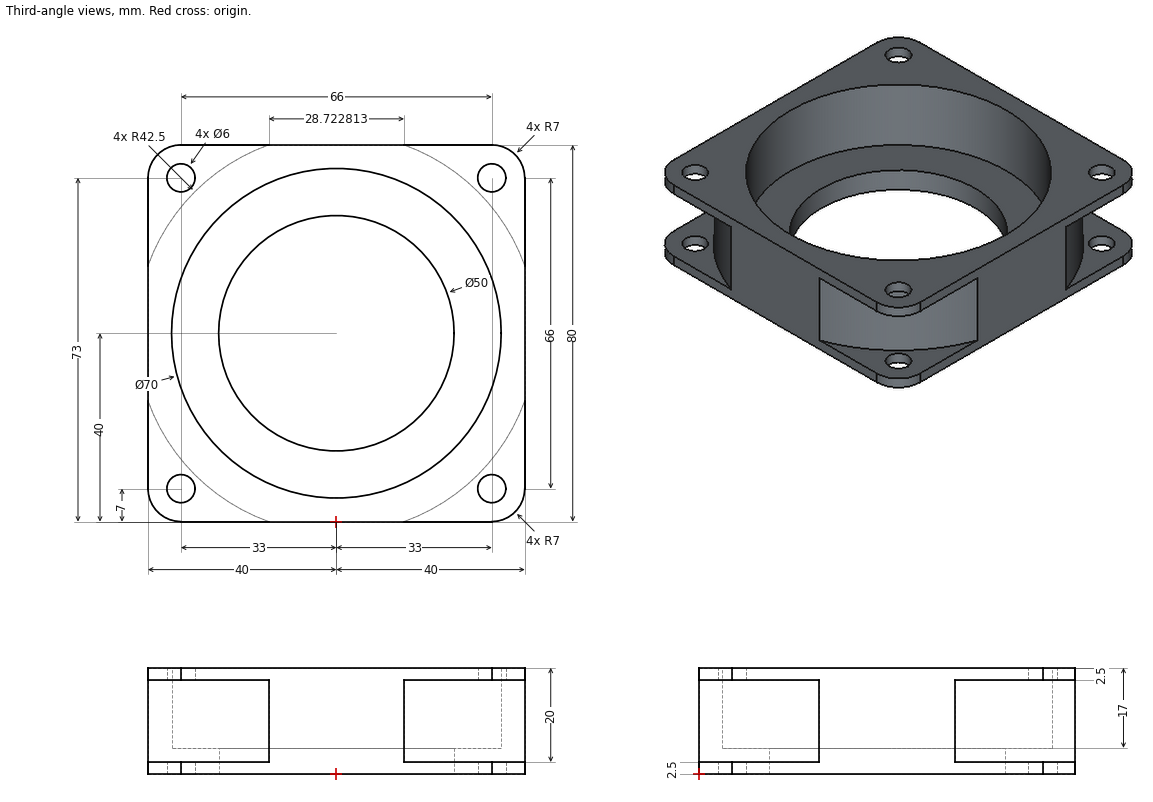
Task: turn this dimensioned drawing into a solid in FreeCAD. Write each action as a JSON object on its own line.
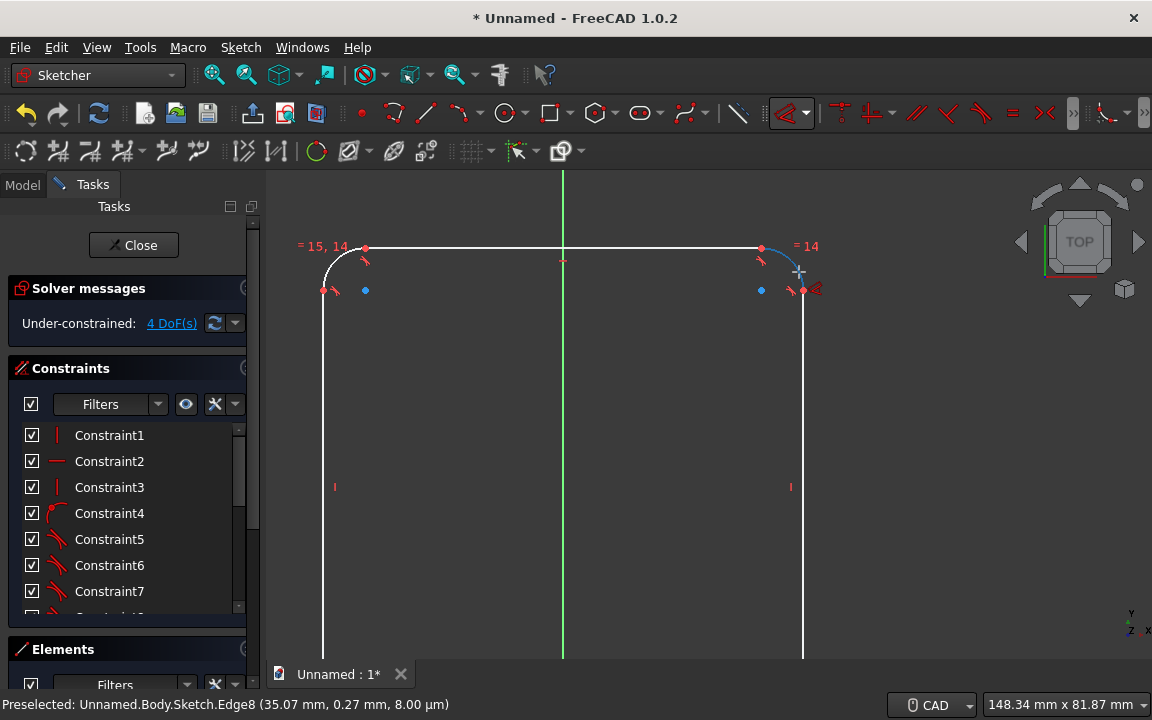
{"action": "left_click", "coordinate": [799, 271]}
{"action": "left_click", "coordinate": [827, 256]}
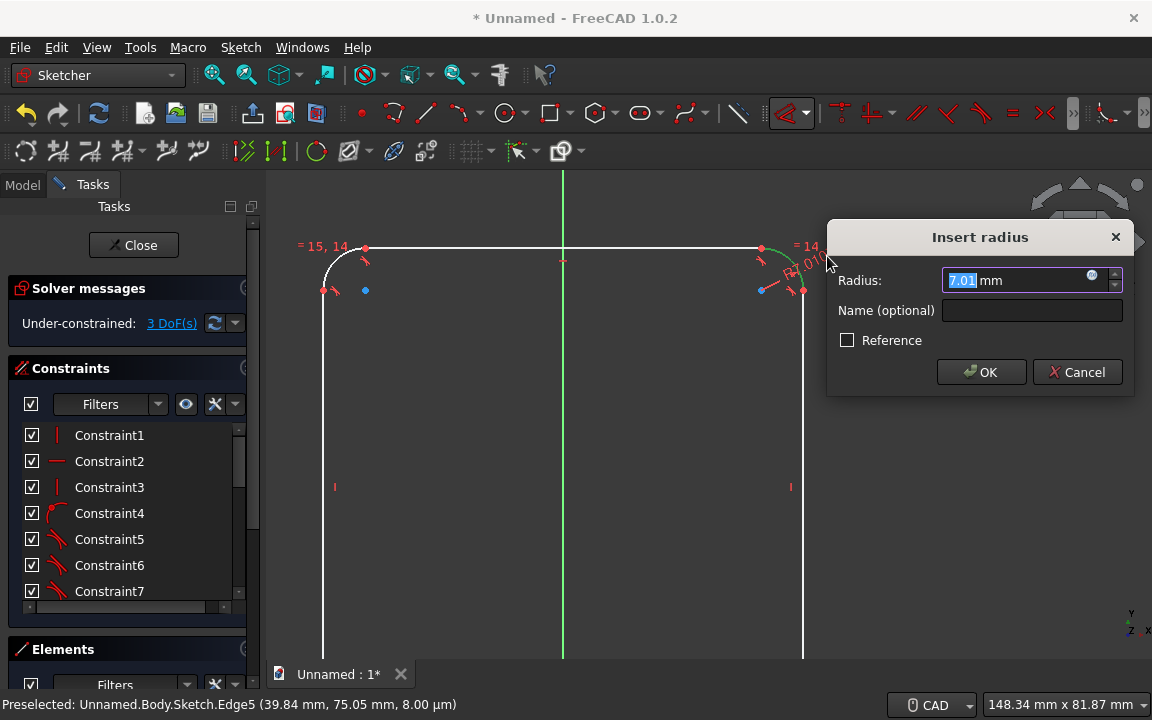
{"action": "type", "text": "7"}
{"action": "key", "text": "Return"}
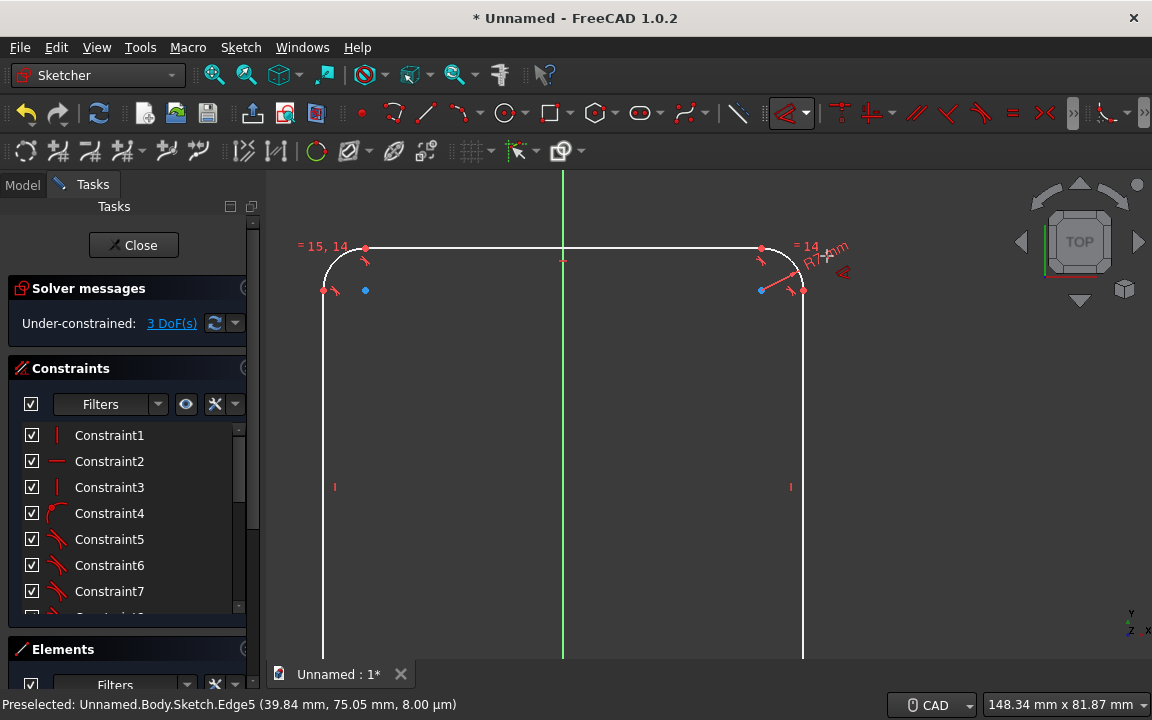
{"action": "left_click", "coordinate": [803, 565]}
{"action": "left_click", "coordinate": [837, 461]}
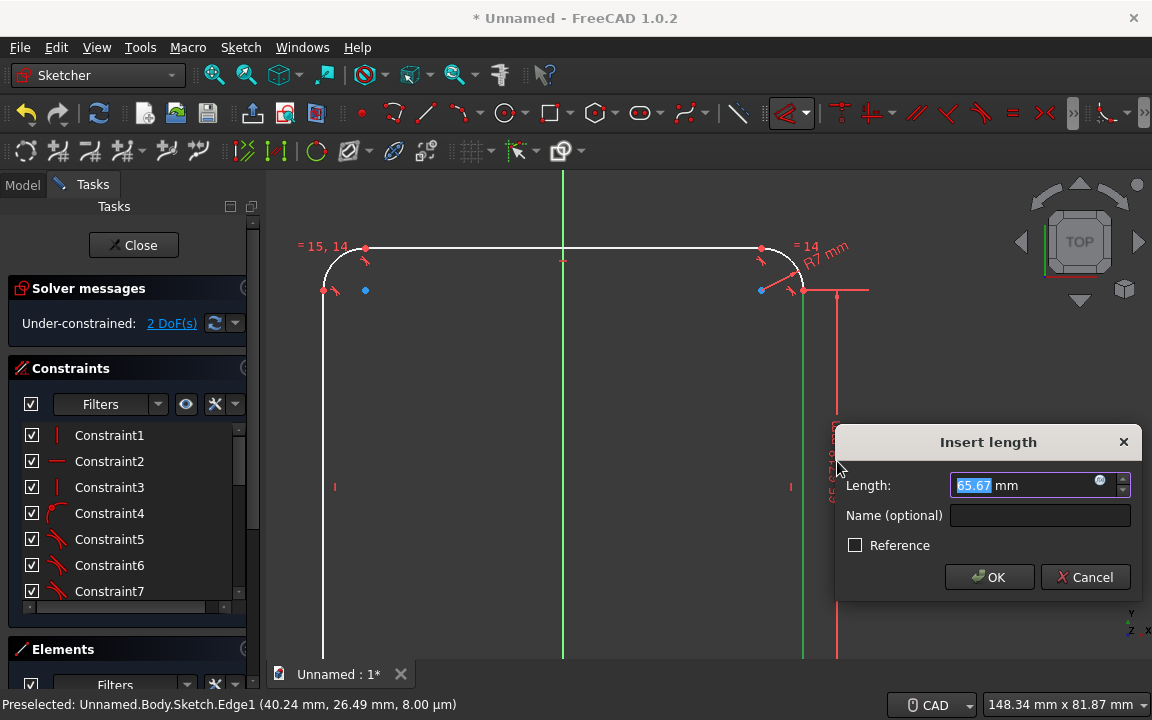
{"action": "type", "text": "66"}
{"action": "key", "text": "Return"}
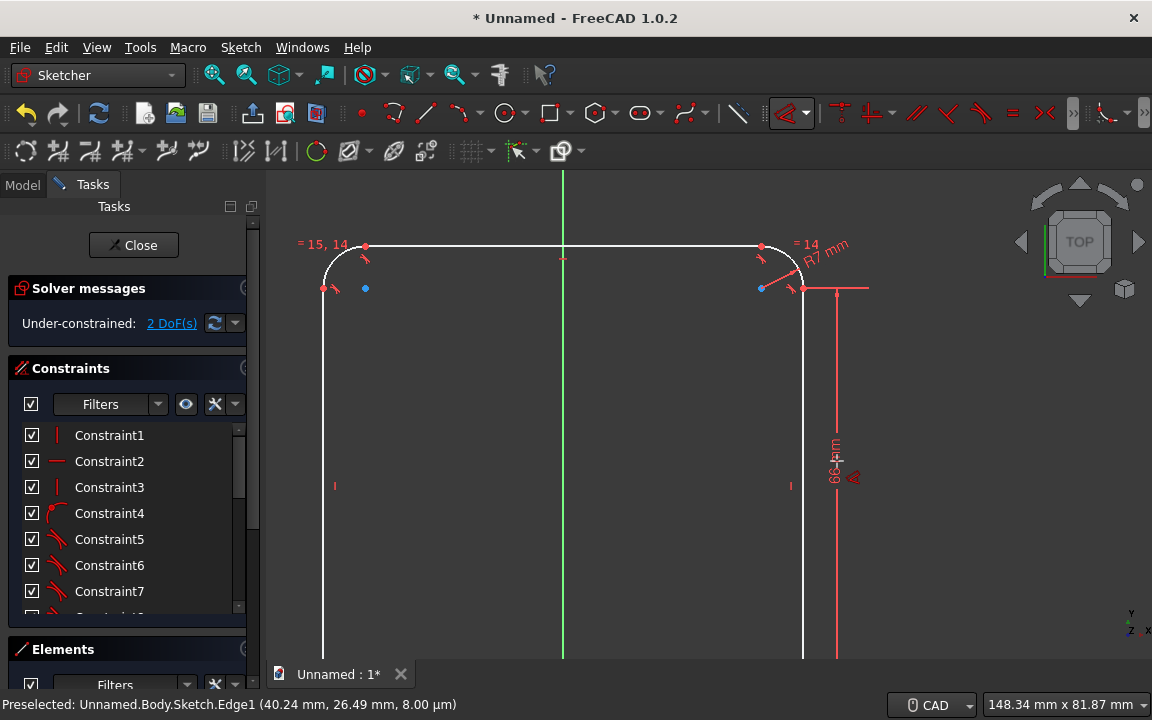
{"action": "left_click", "coordinate": [643, 246]}
{"action": "left_click", "coordinate": [472, 212]}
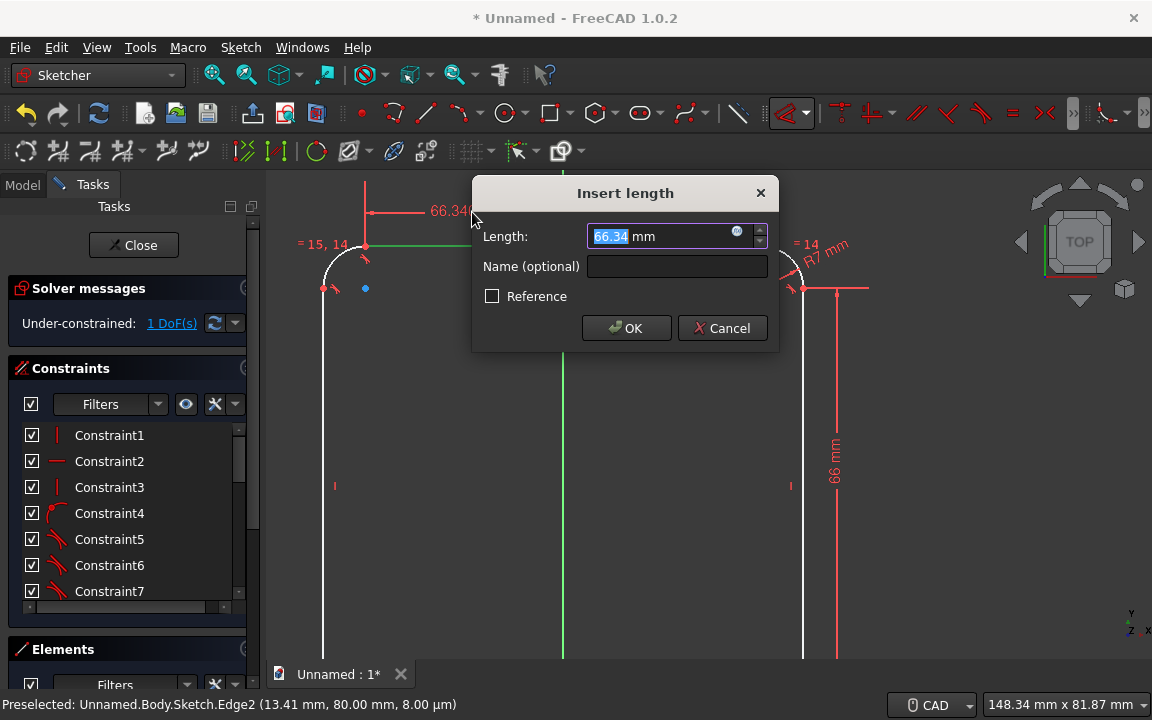
{"action": "type", "text": "66"}
{"action": "key", "text": "Return"}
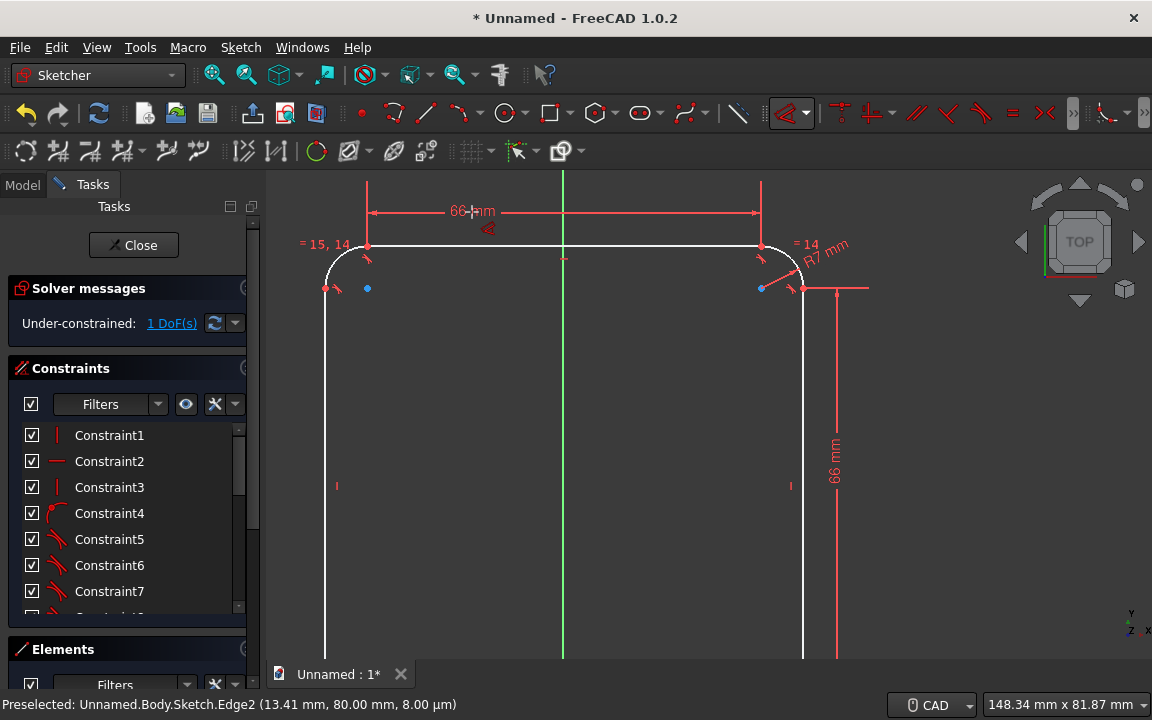
{"action": "scroll", "coordinate": [798, 270], "scroll_direction": "down", "scroll_amount": 2}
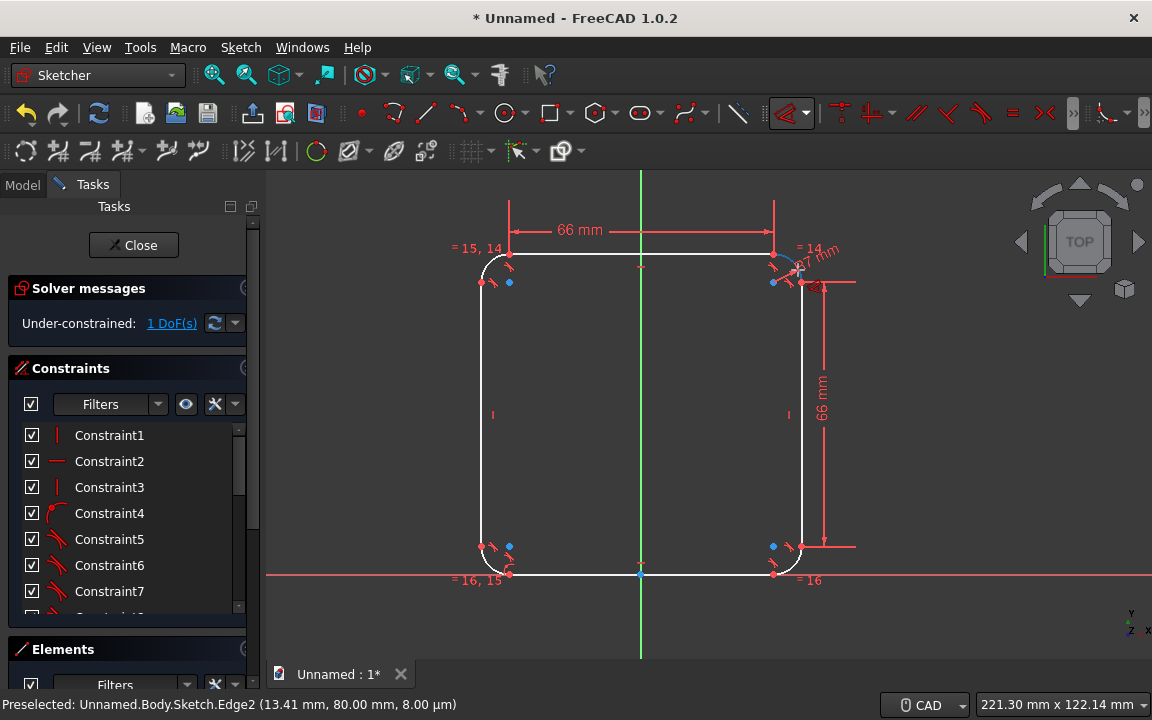
{"action": "left_click", "coordinate": [802, 547]}
{"action": "left_click", "coordinate": [721, 609]}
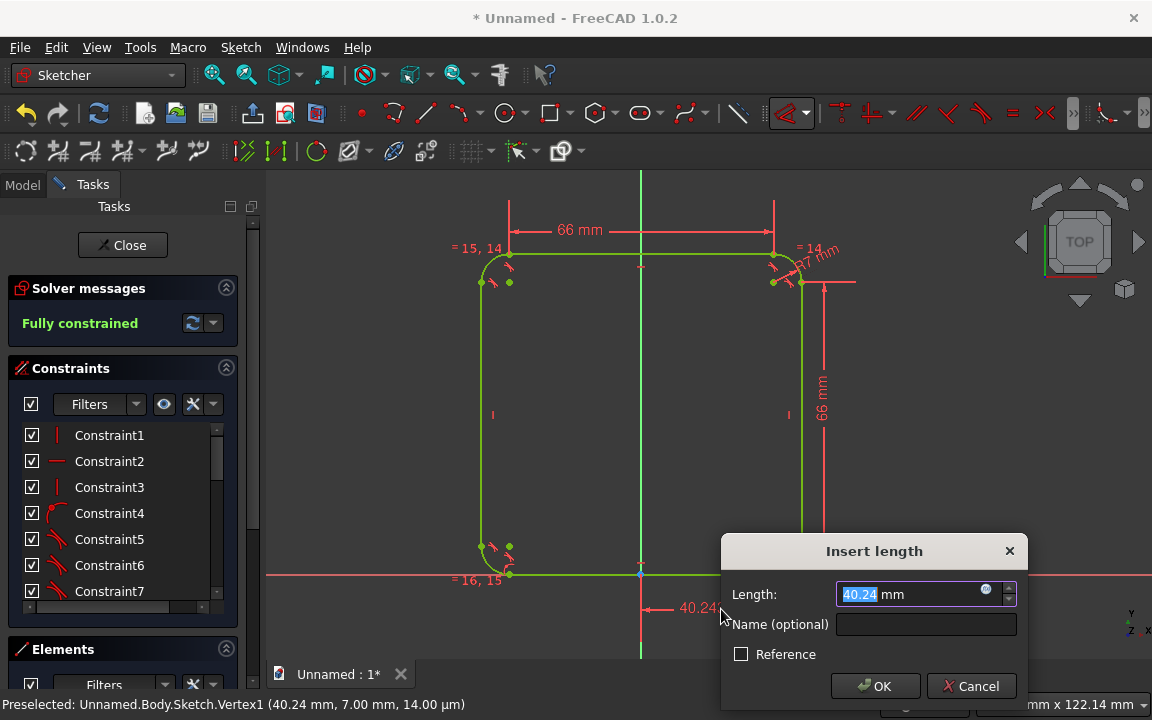
{"action": "type", "text": "40"}
{"action": "key", "text": "Return"}
{"action": "key", "text": "Escape"}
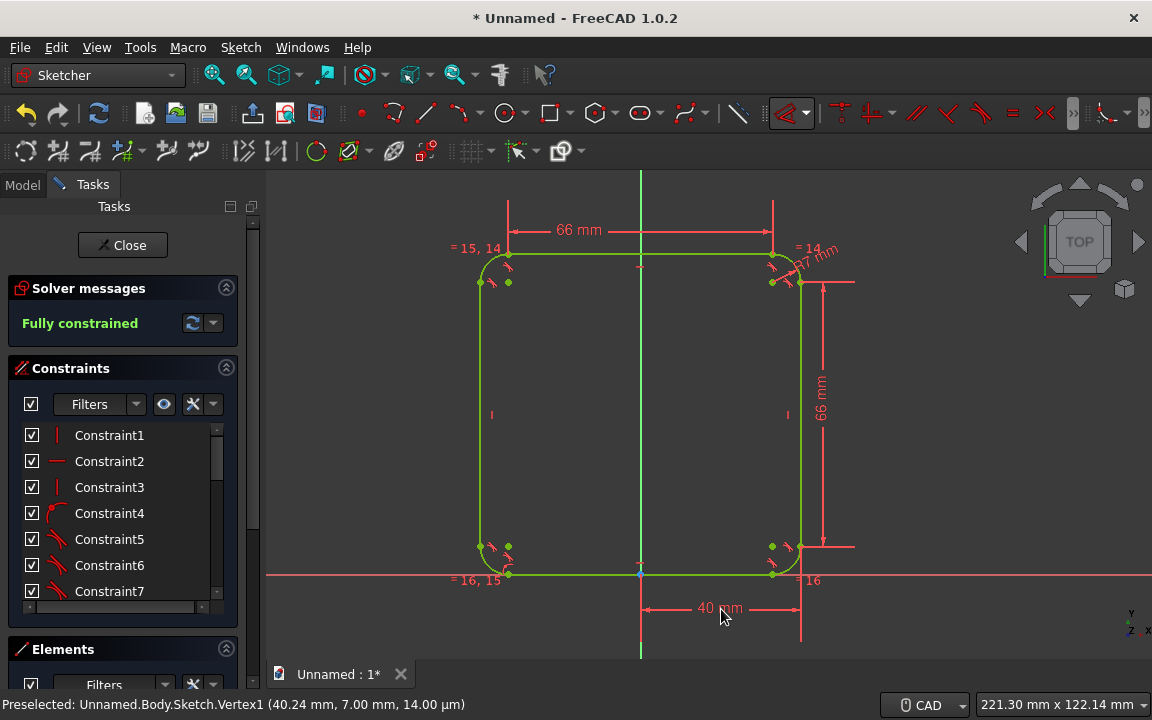
{"action": "left_click", "coordinate": [123, 245]}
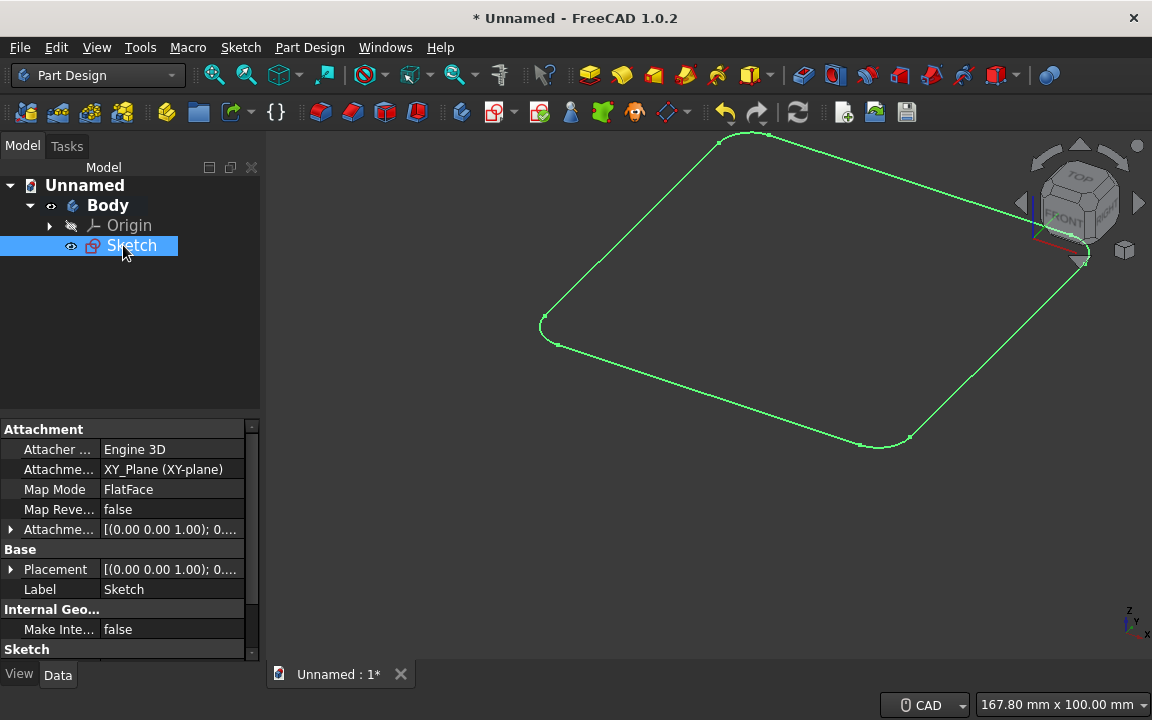
{"action": "left_click", "coordinate": [590, 76]}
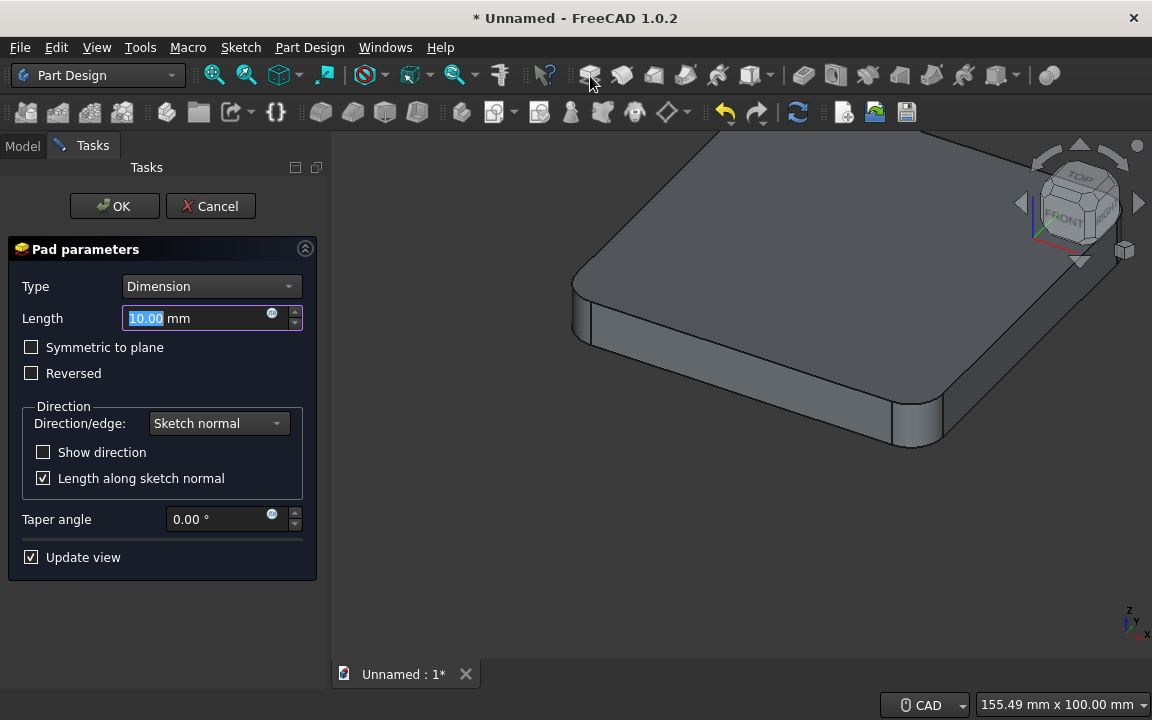
{"action": "type", "text": "2.5"}
{"action": "key", "text": "Tab"}